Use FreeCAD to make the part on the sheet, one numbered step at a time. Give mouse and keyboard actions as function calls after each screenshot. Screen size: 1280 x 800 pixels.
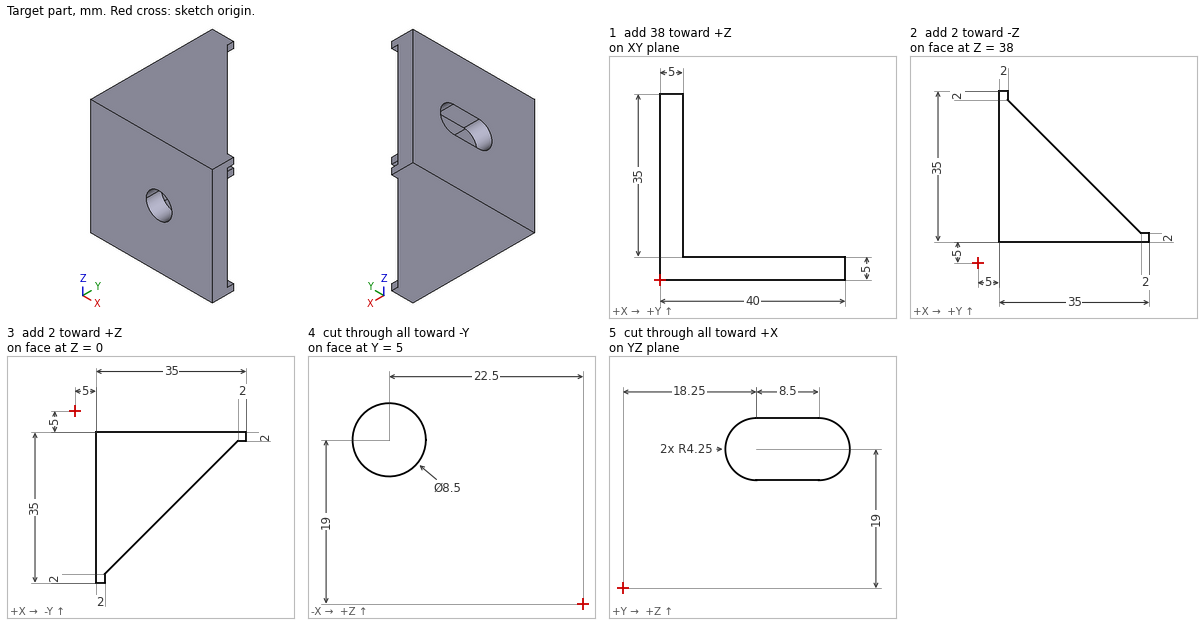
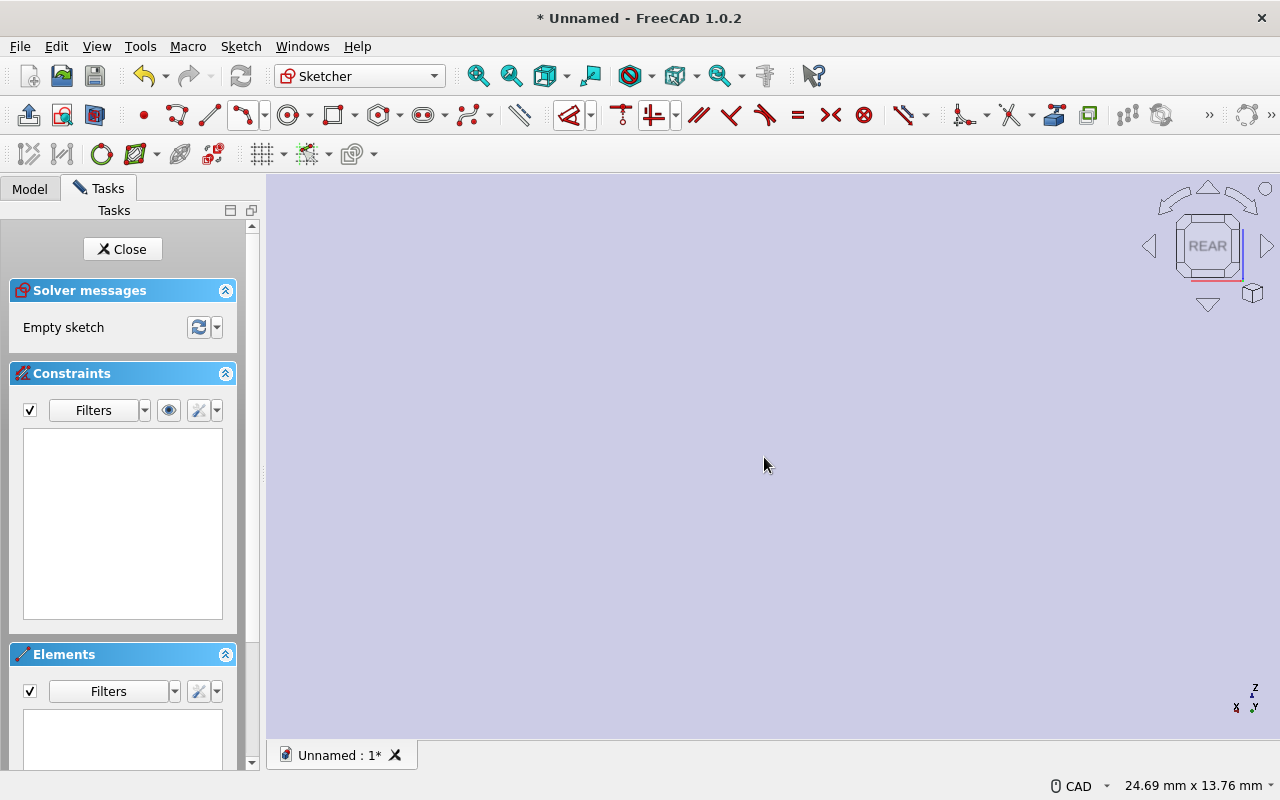
key(g)
key(c)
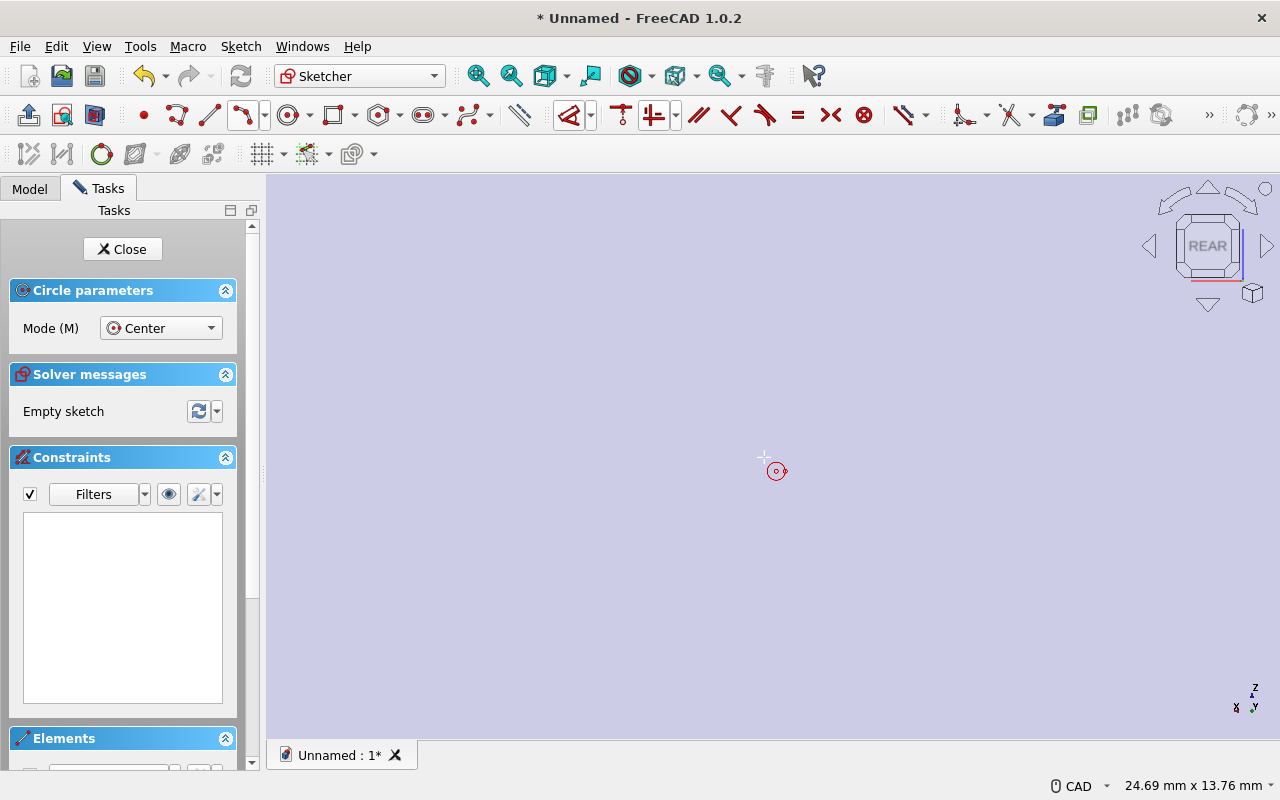
click(704, 453)
click(827, 329)
key(Escape)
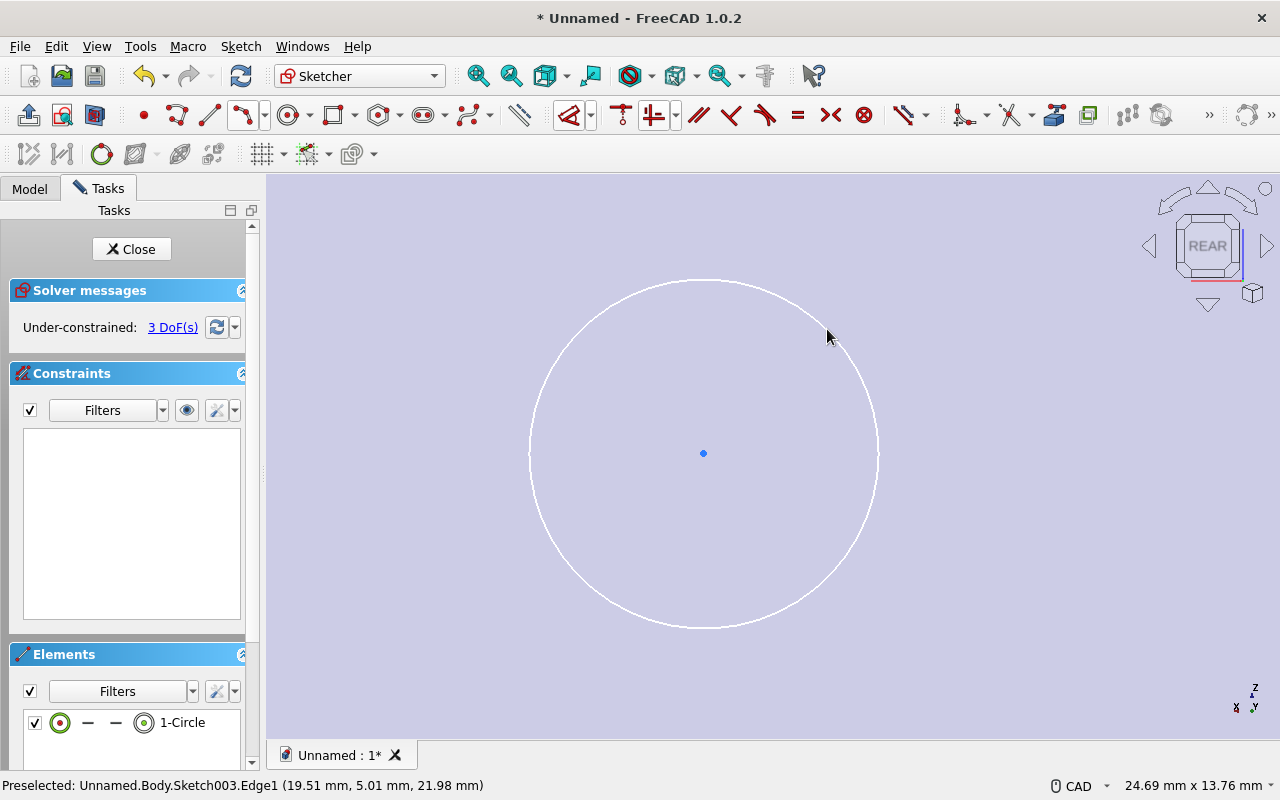
click(827, 330)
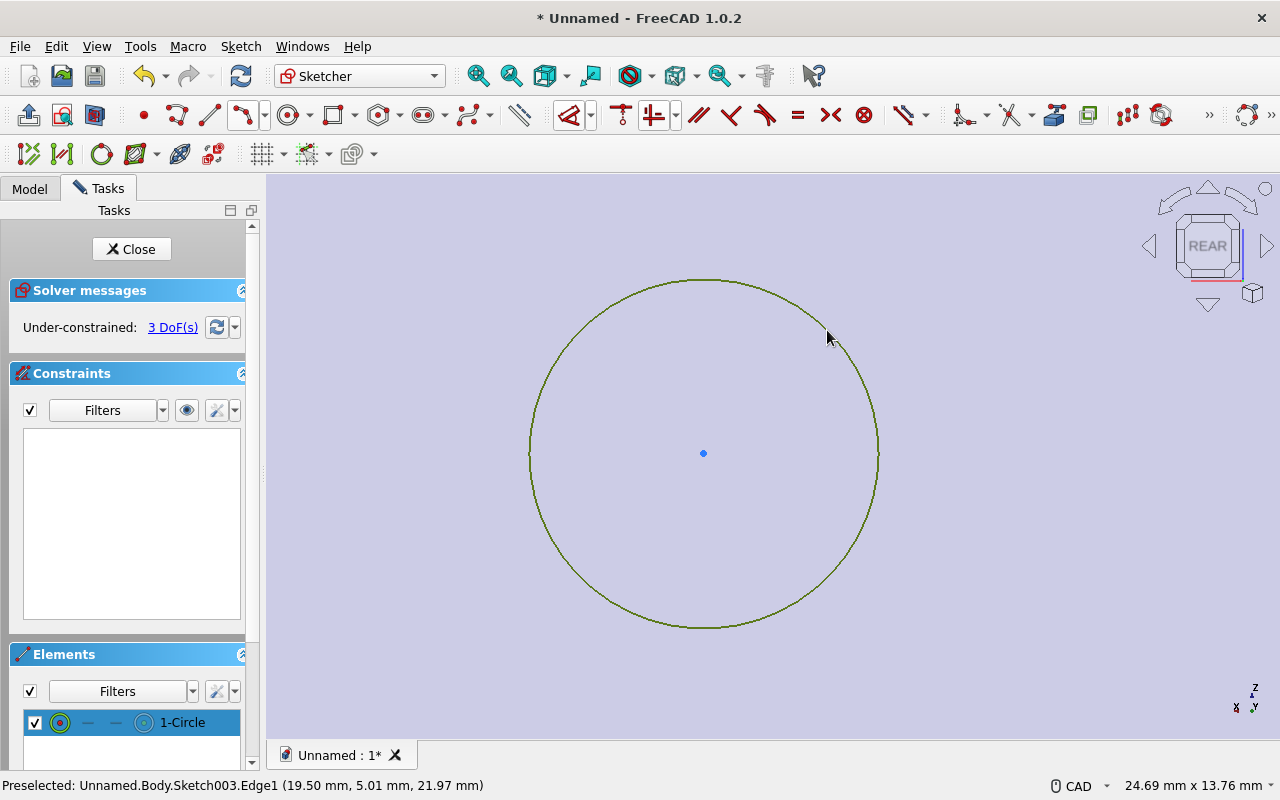
key(k)
key(o)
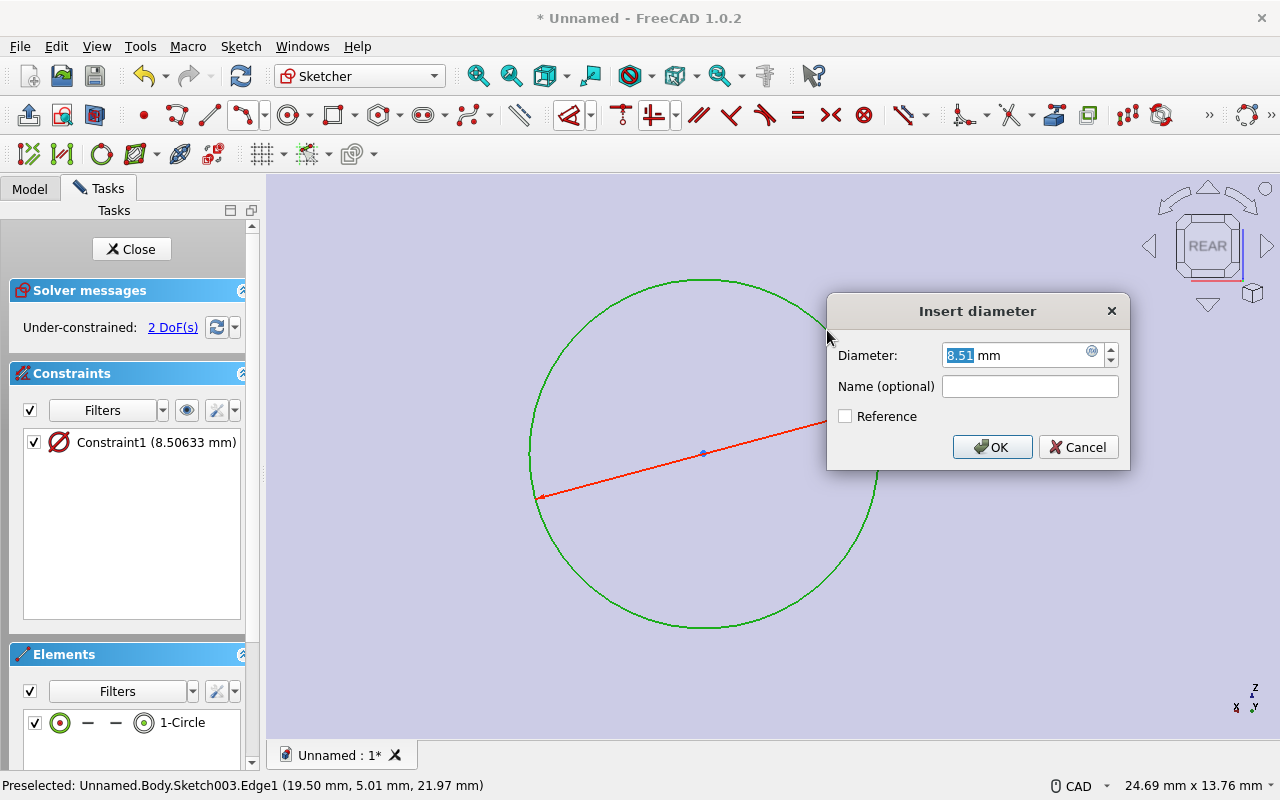
text(8.5)
key(Return)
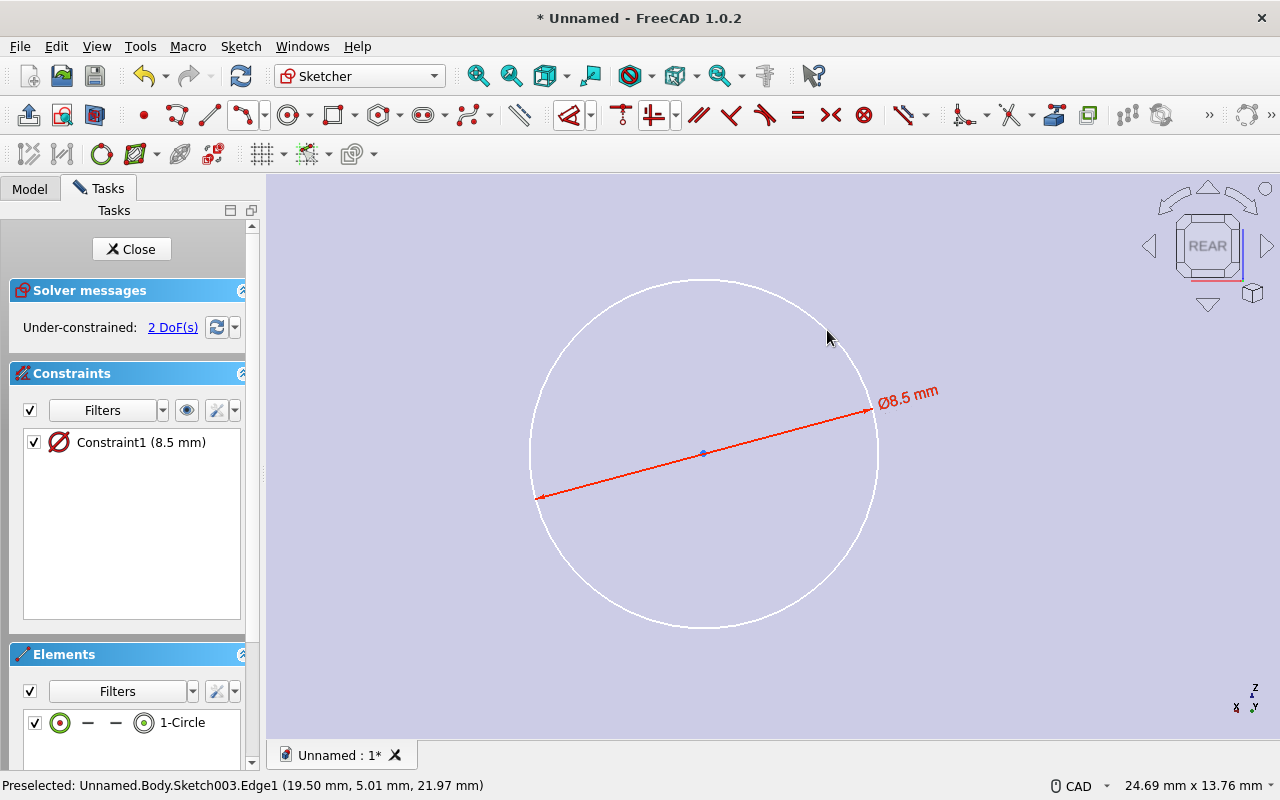
click(704, 454)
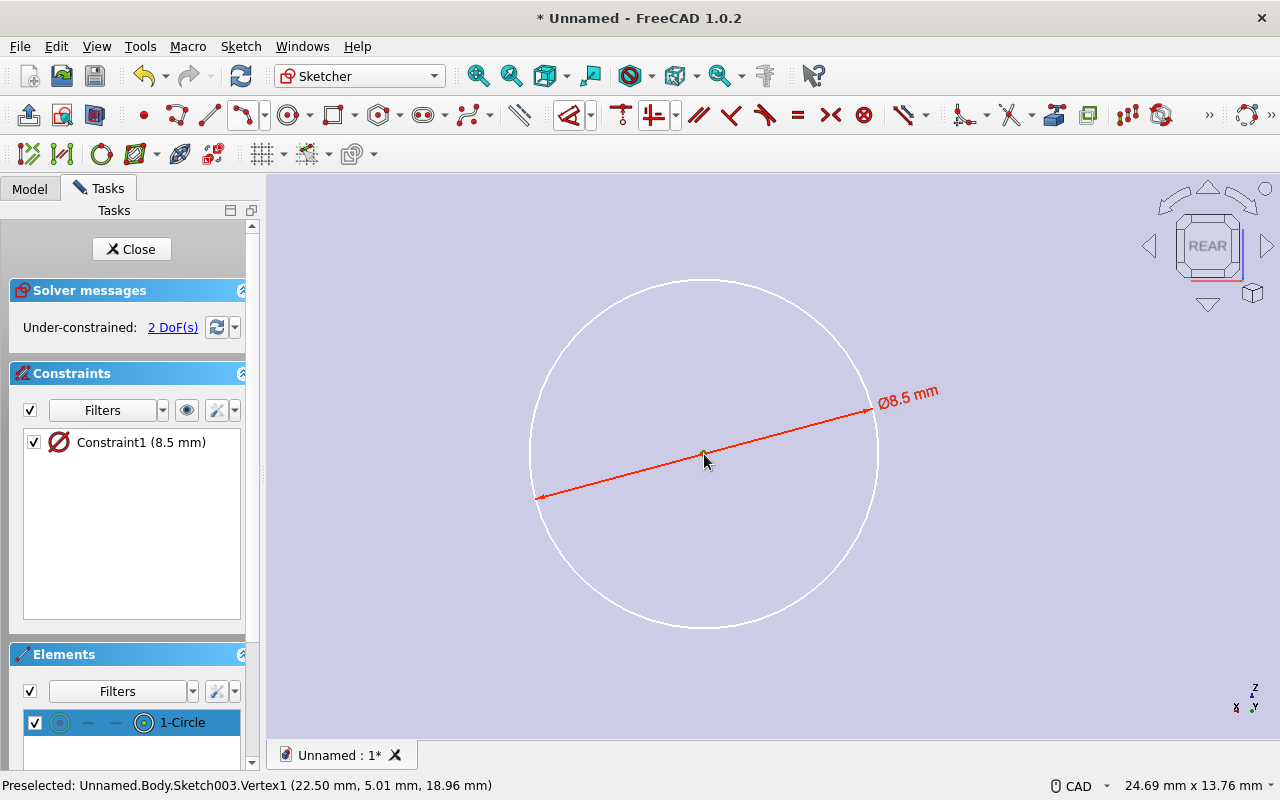
key(i)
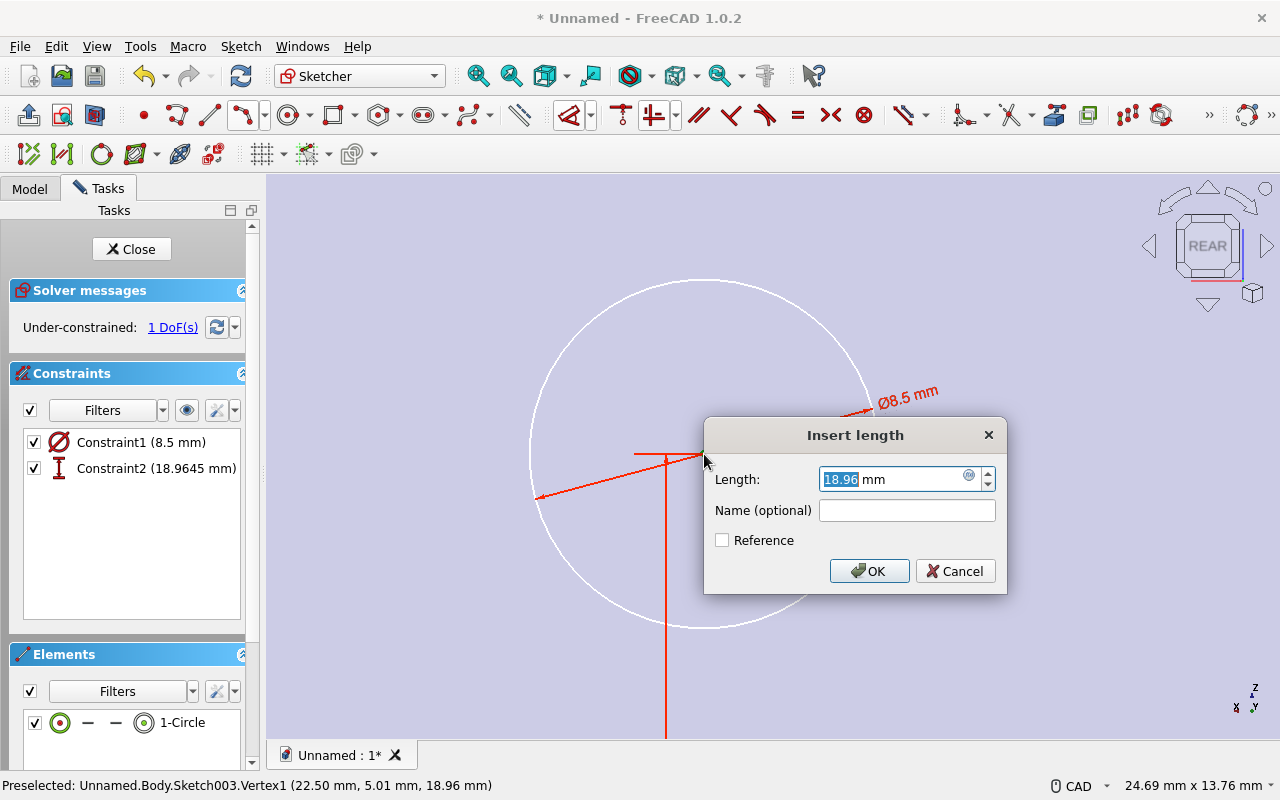
text(19)
key(Return)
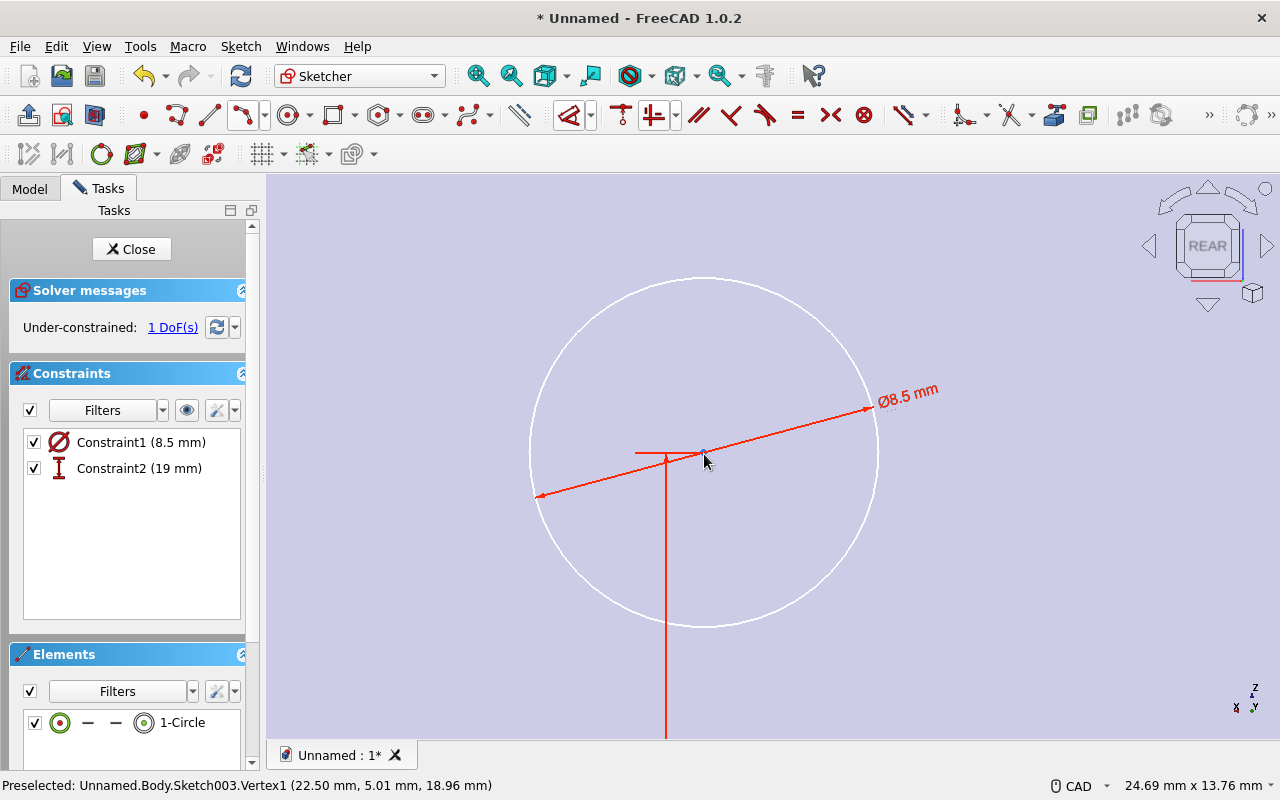
click(704, 453)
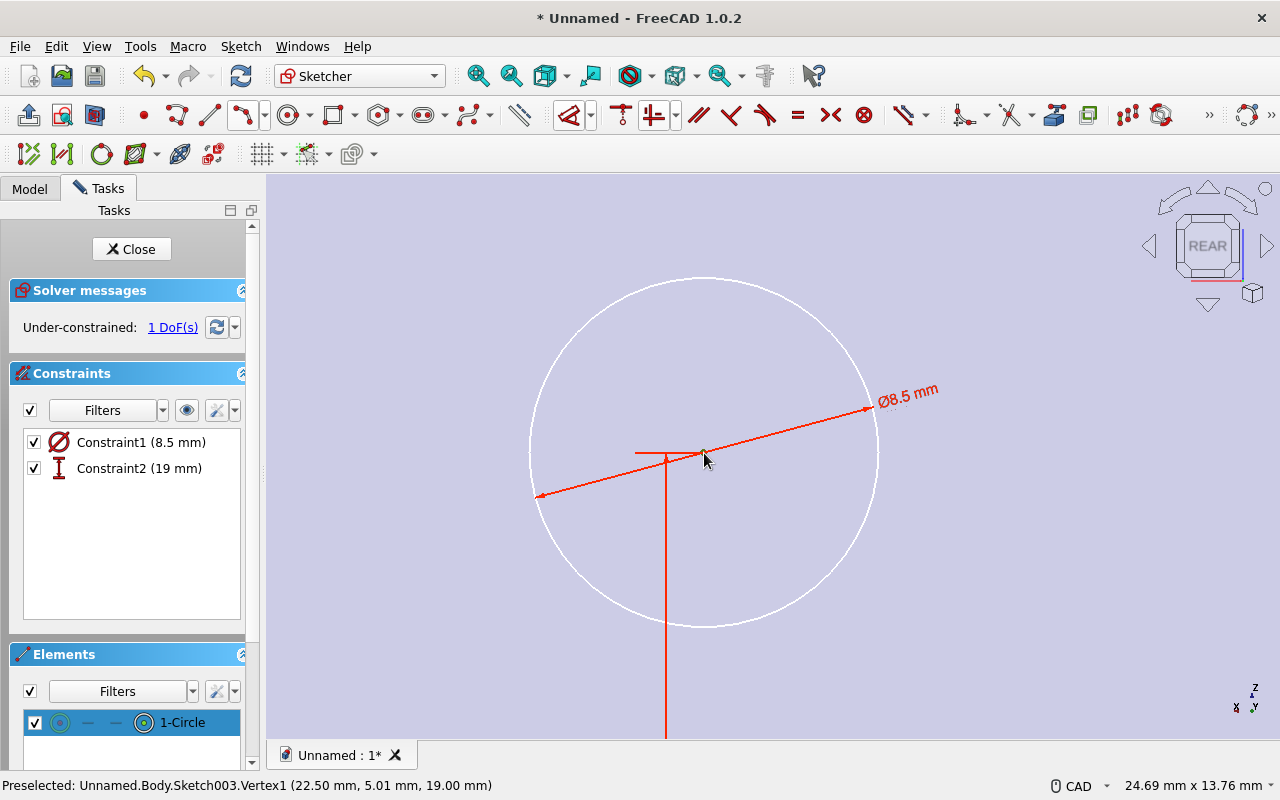
key(l)